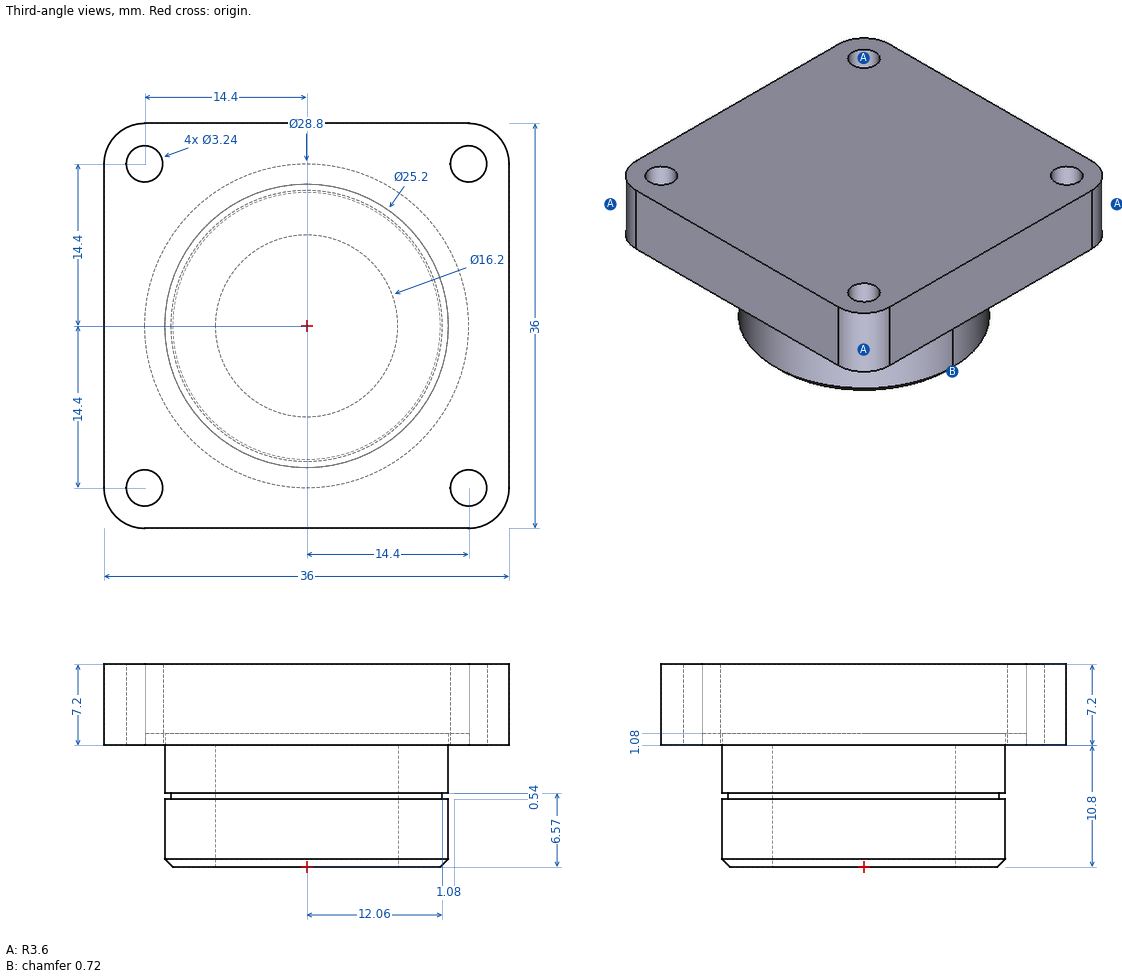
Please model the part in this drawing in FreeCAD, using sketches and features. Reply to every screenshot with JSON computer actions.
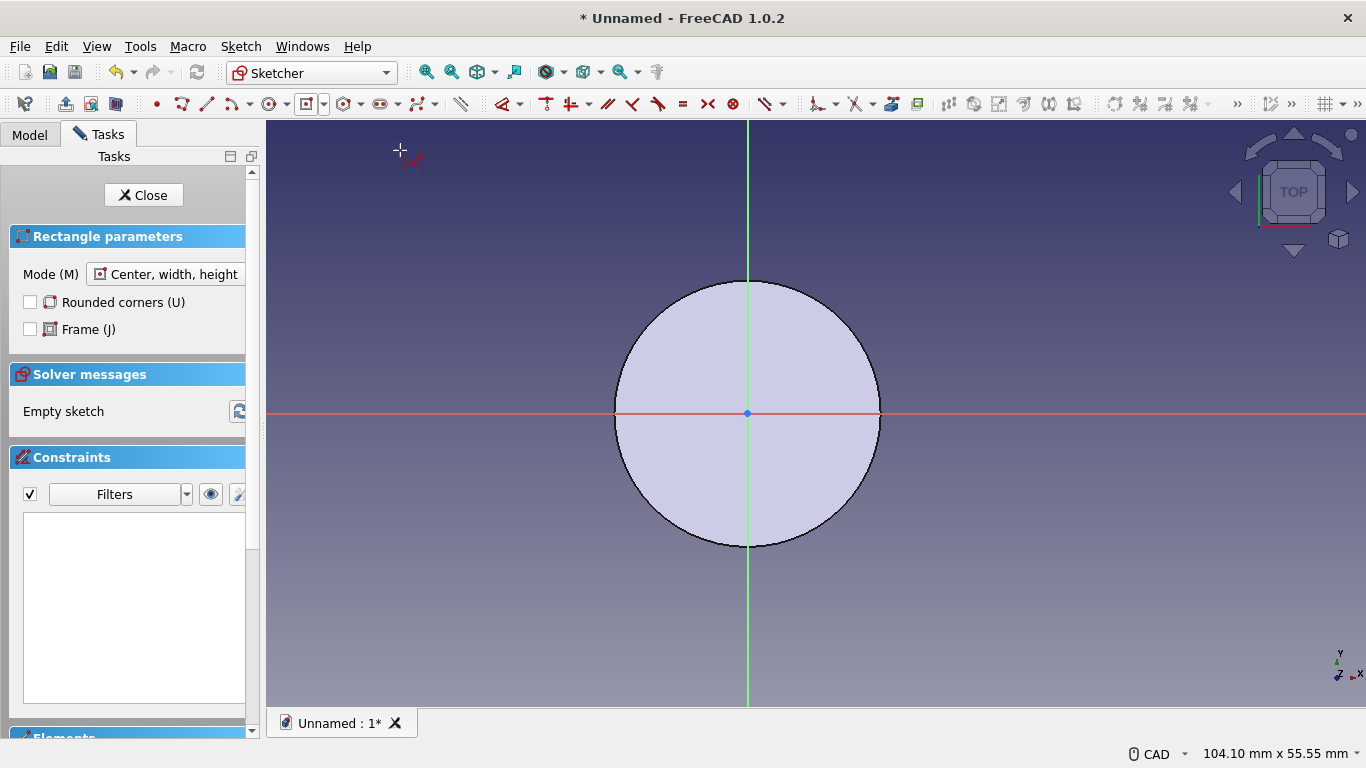
{"action": "left_click", "coordinate": [748, 414]}
{"action": "mouse_move", "coordinate": [938, 224]}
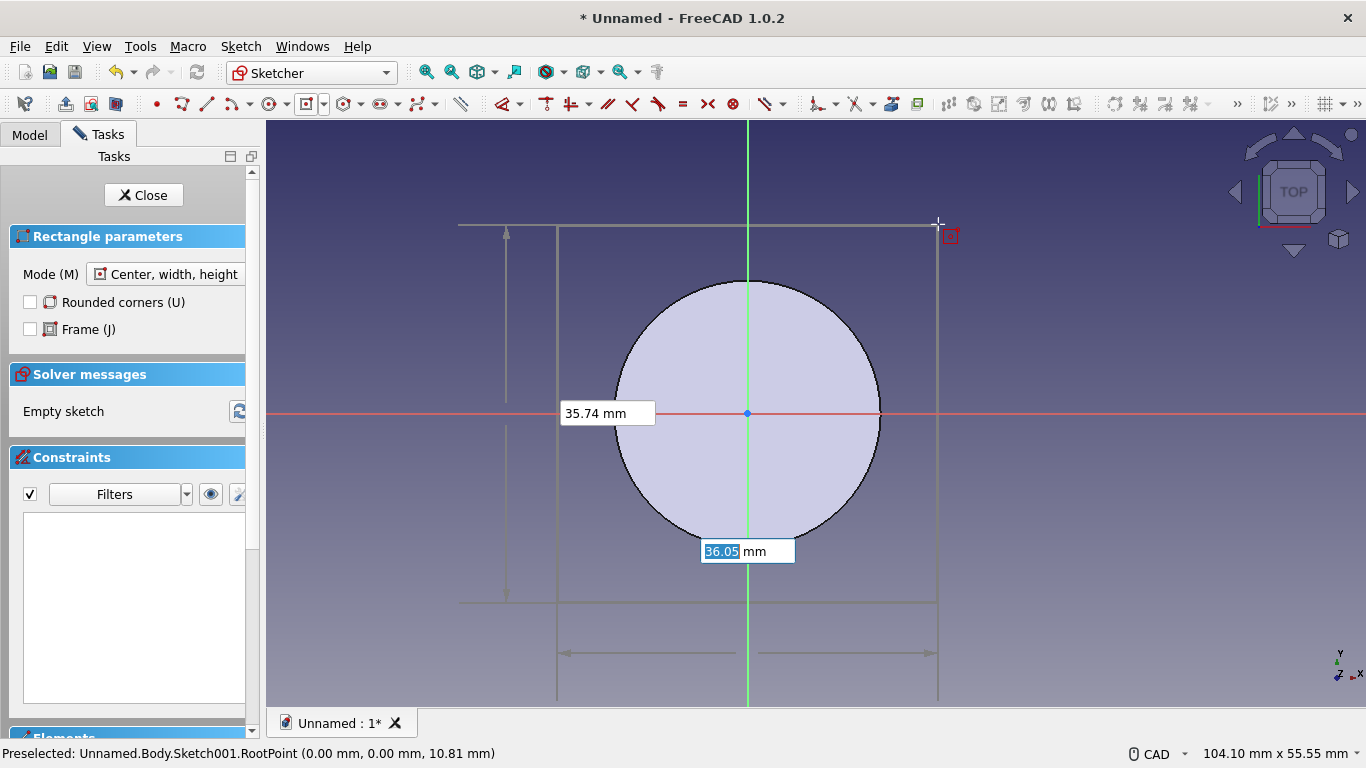
{"action": "type", "text": "36"}
{"action": "key", "text": "Tab"}
{"action": "type", "text": "36"}
{"action": "key", "text": "Return"}
{"action": "key", "text": "Escape"}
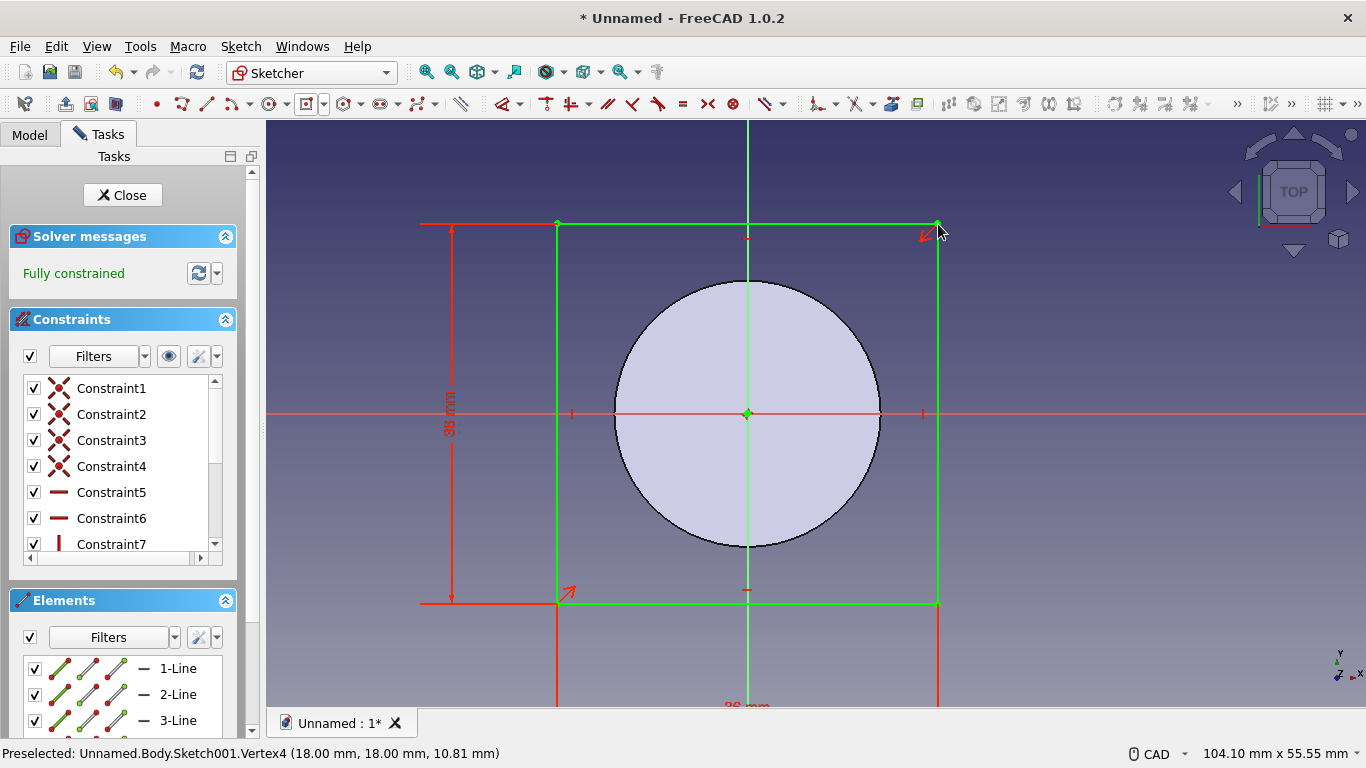
{"action": "left_click", "coordinate": [123, 195]}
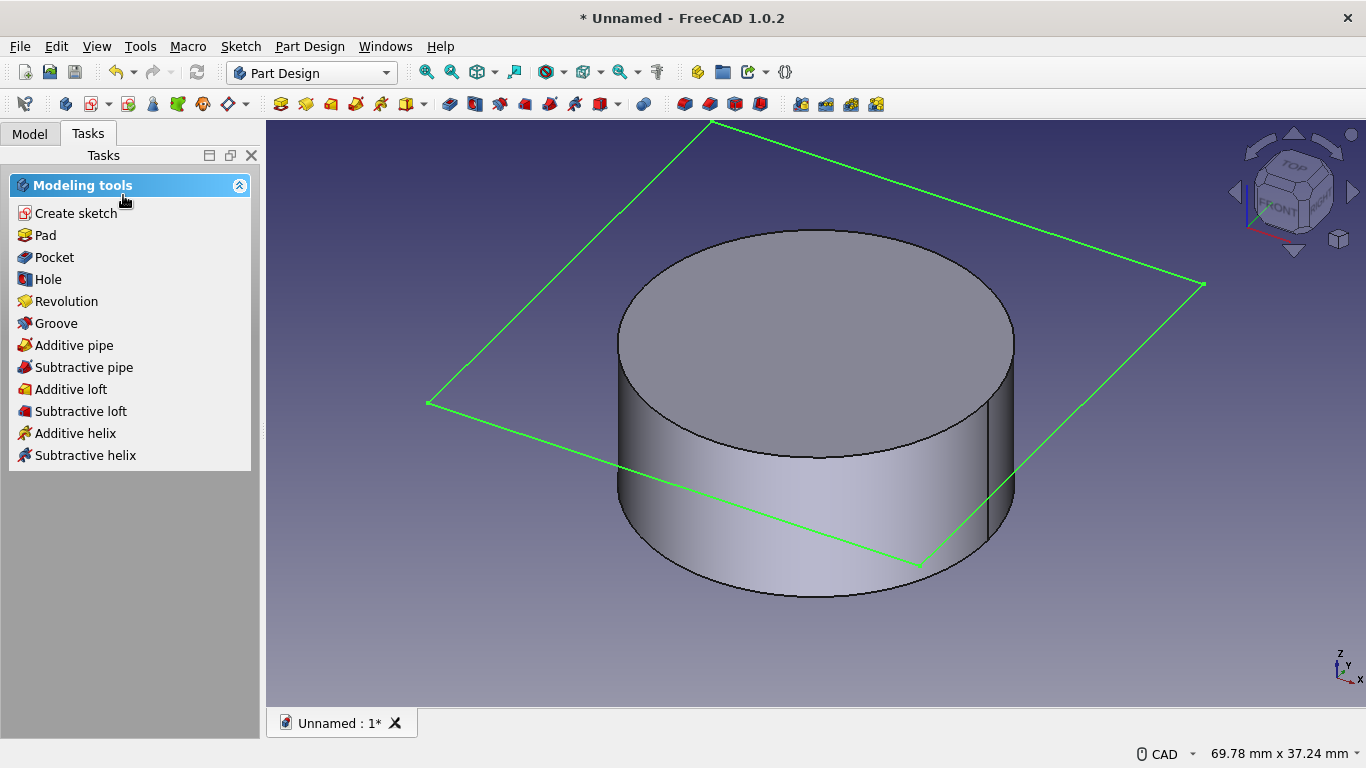
{"action": "left_click", "coordinate": [281, 104]}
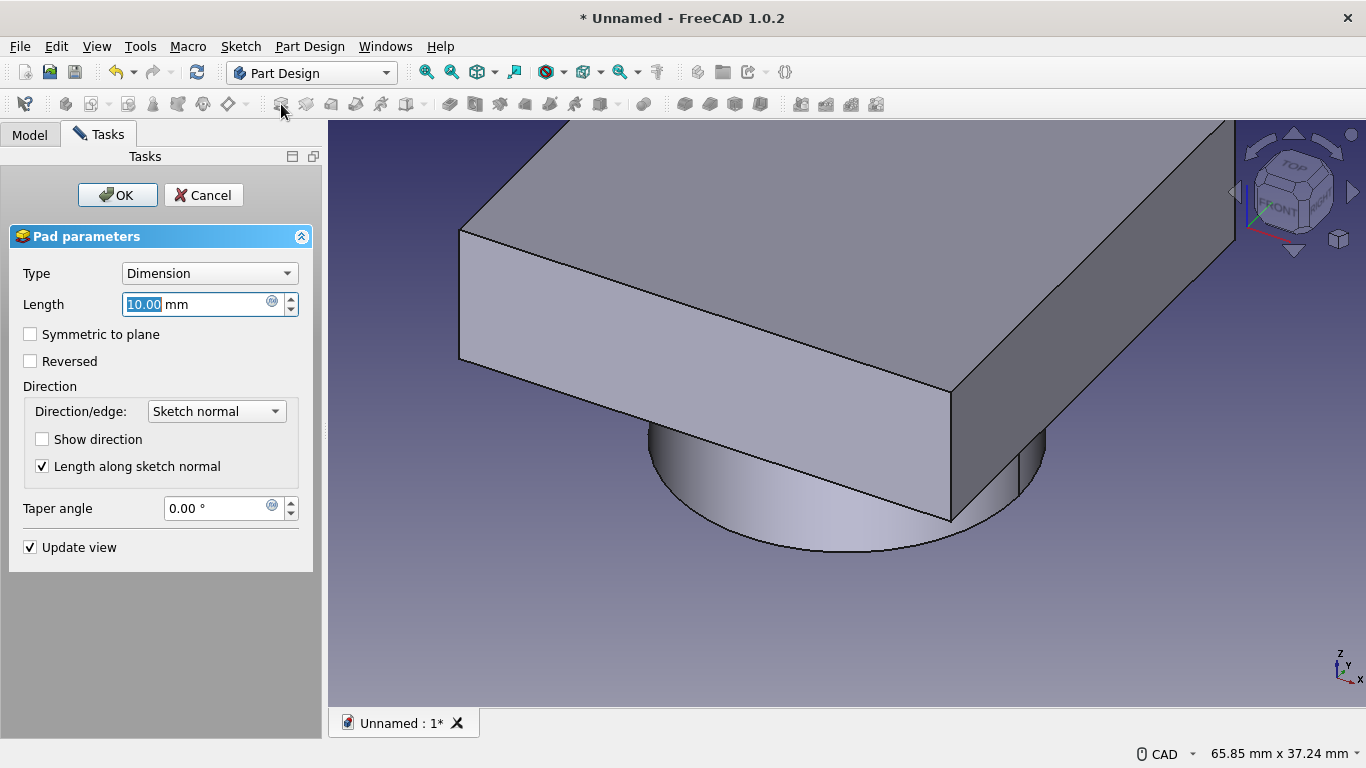
{"action": "type", "text": "7.2"}
{"action": "key", "text": "Tab"}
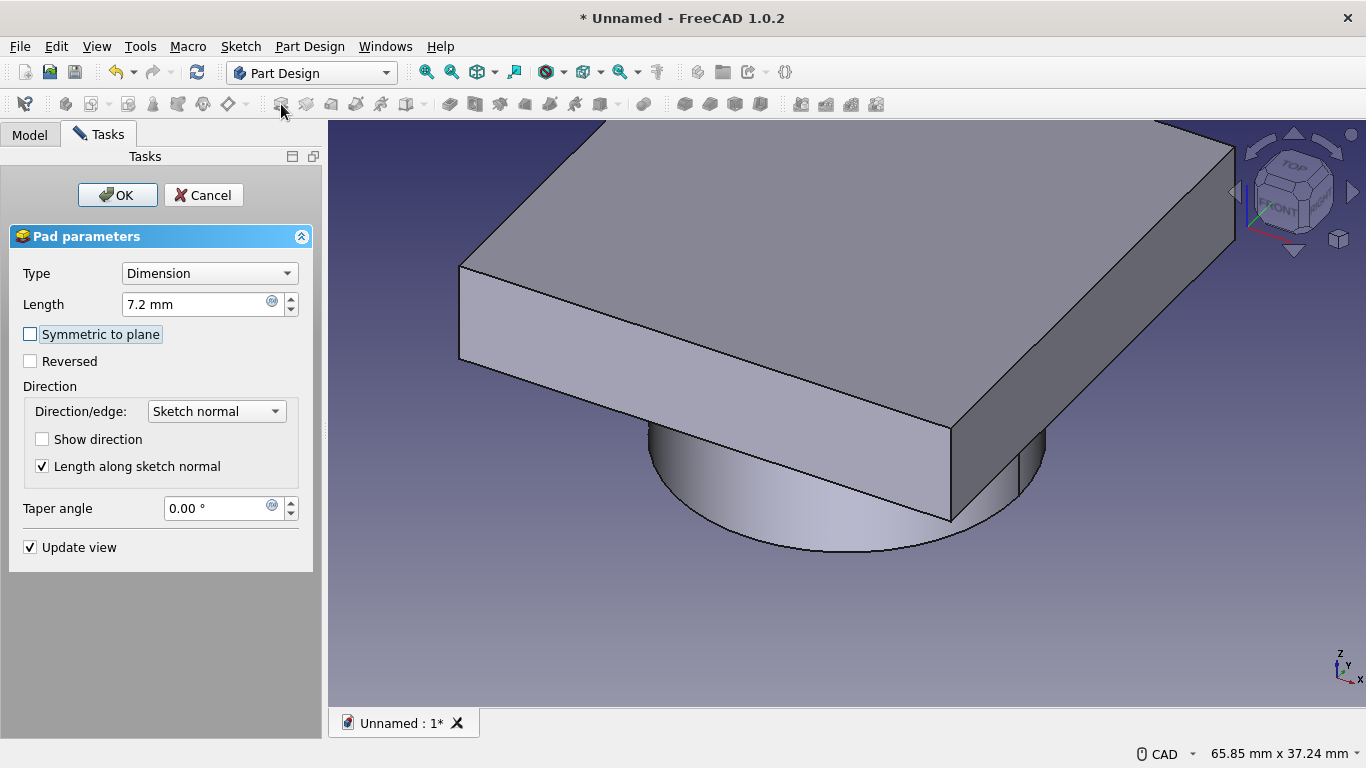
{"action": "left_click", "coordinate": [118, 195]}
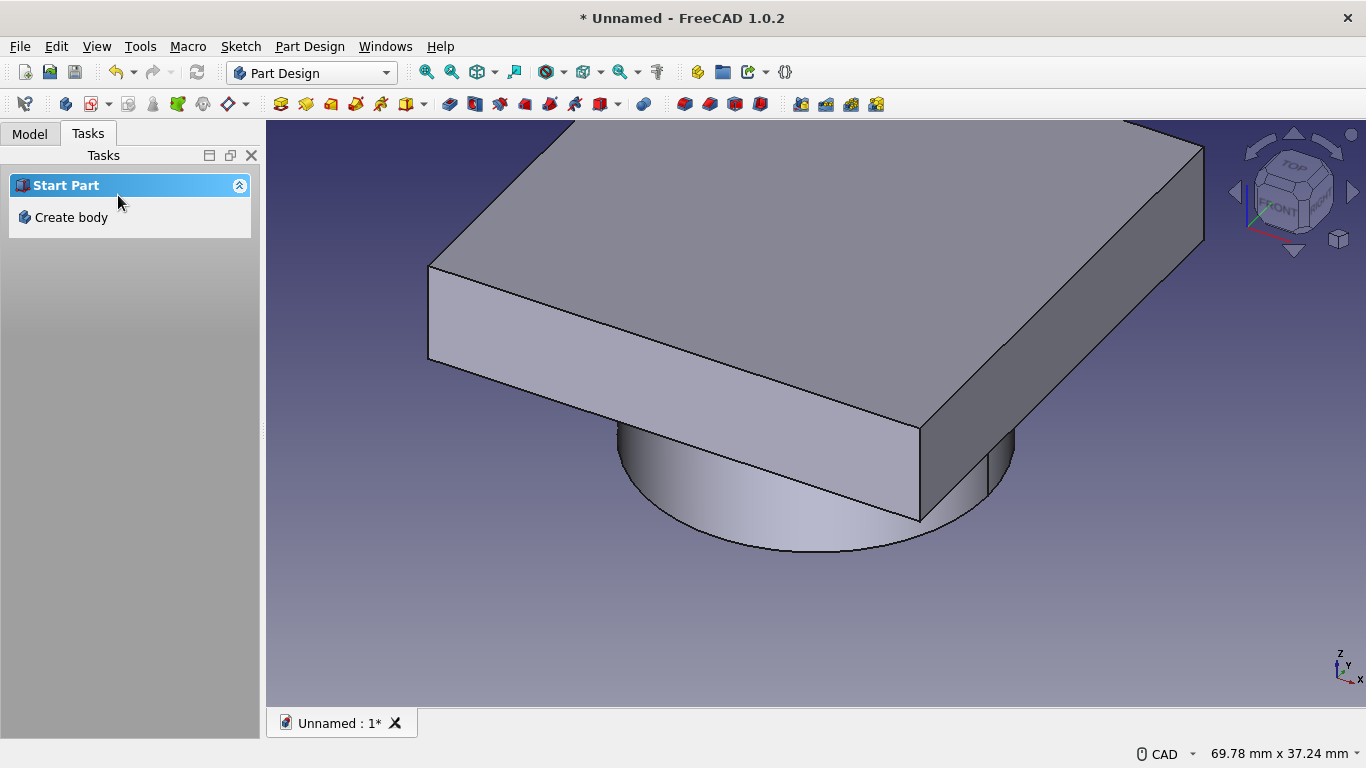
{"action": "left_click", "coordinate": [427, 72]}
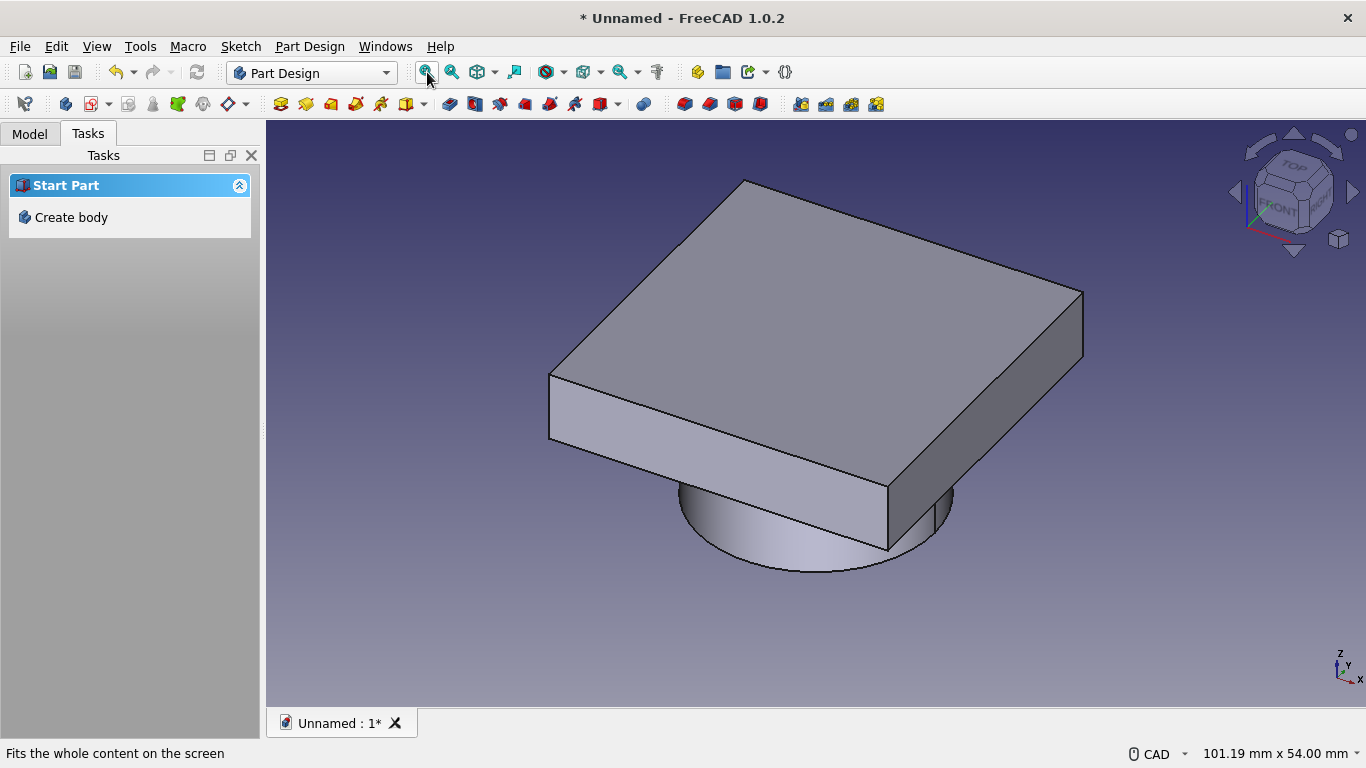
{"action": "left_click", "coordinate": [888, 518]}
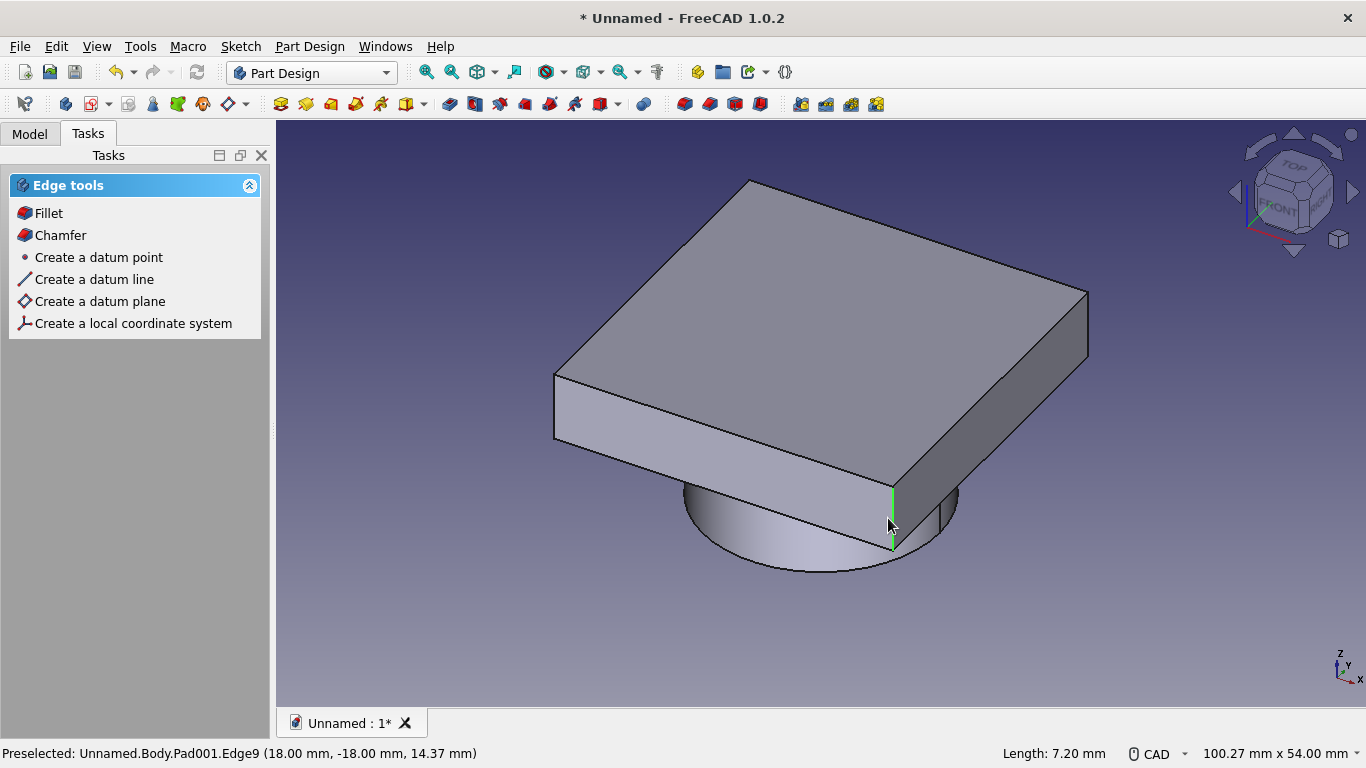
{"action": "key", "text": "0"}